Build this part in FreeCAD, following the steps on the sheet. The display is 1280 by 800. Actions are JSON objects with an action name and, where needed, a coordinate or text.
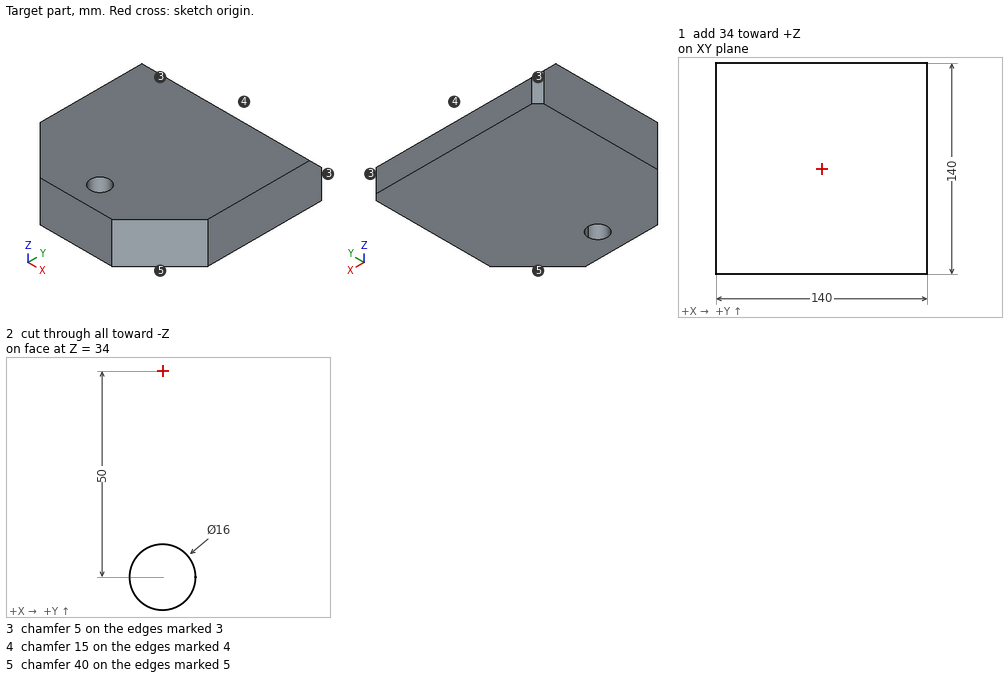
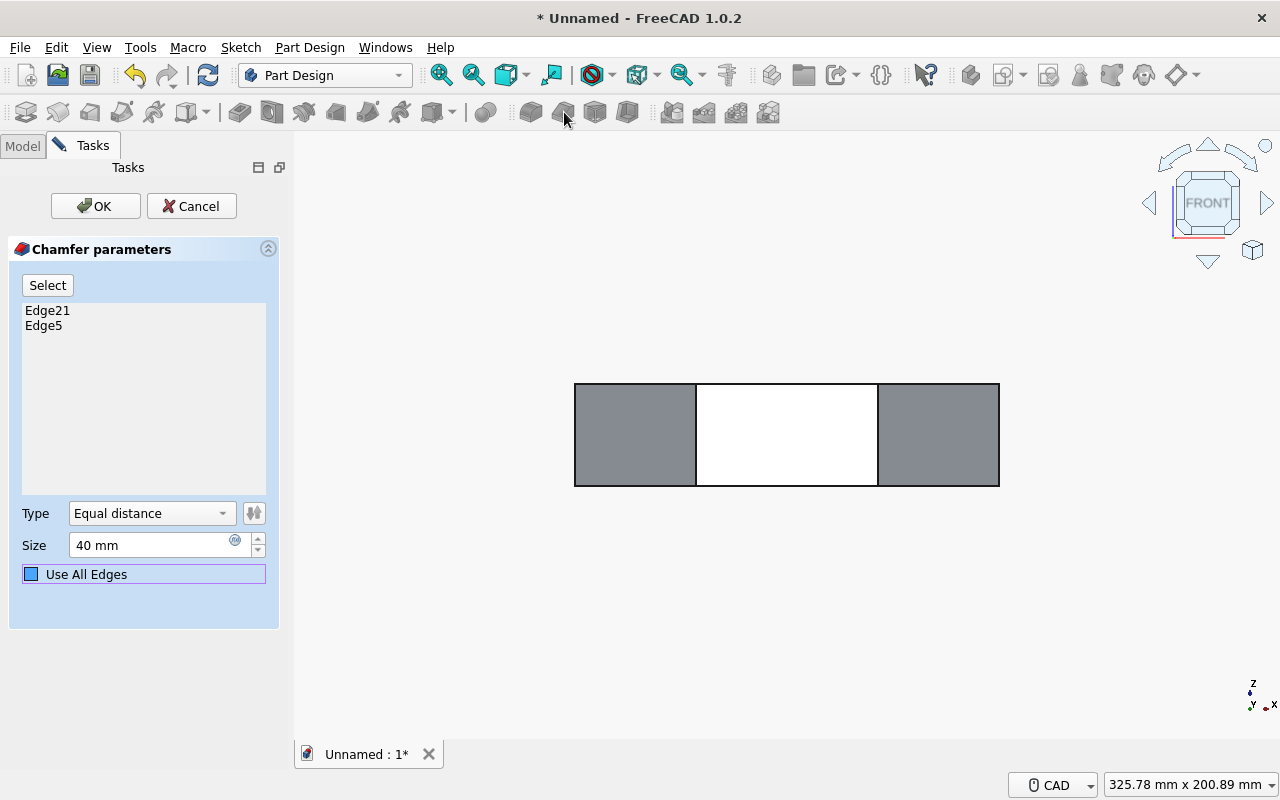
{"action": "left_click", "coordinate": [96, 206]}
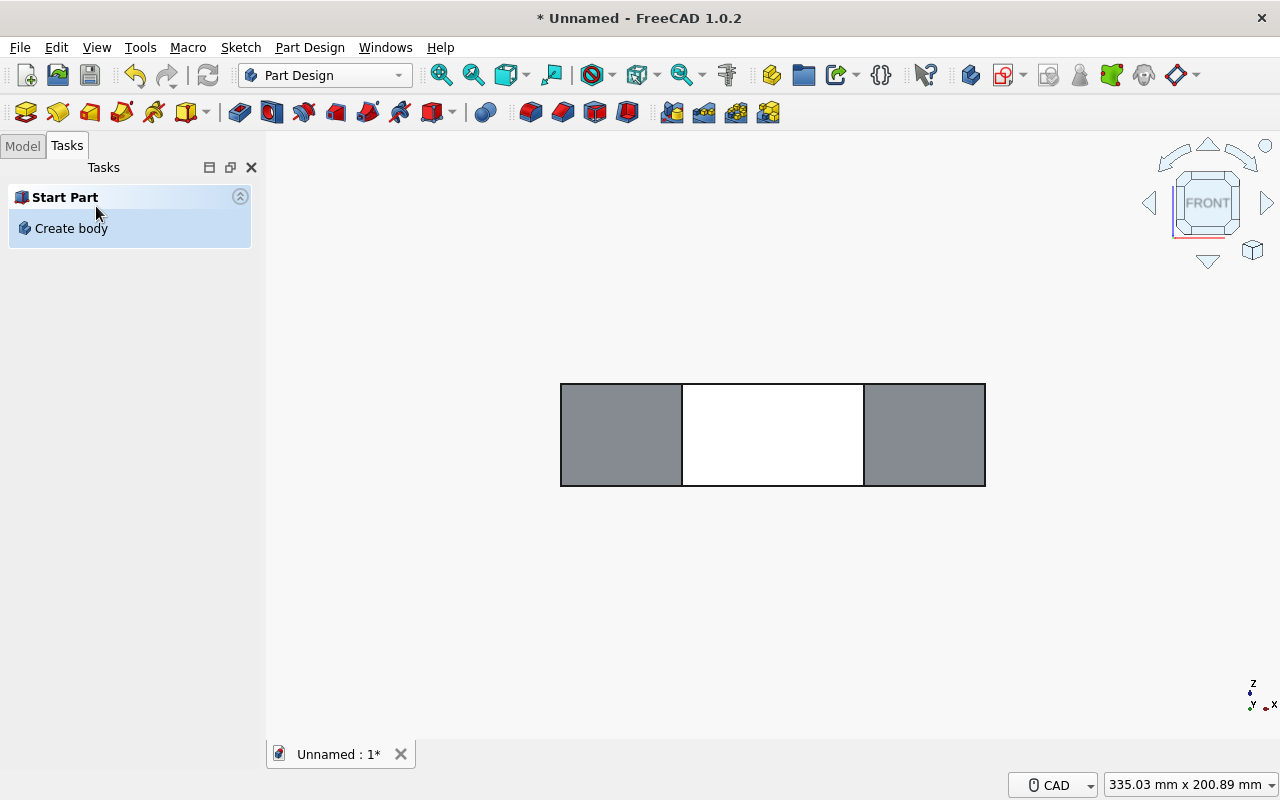
{"action": "key", "text": "0"}